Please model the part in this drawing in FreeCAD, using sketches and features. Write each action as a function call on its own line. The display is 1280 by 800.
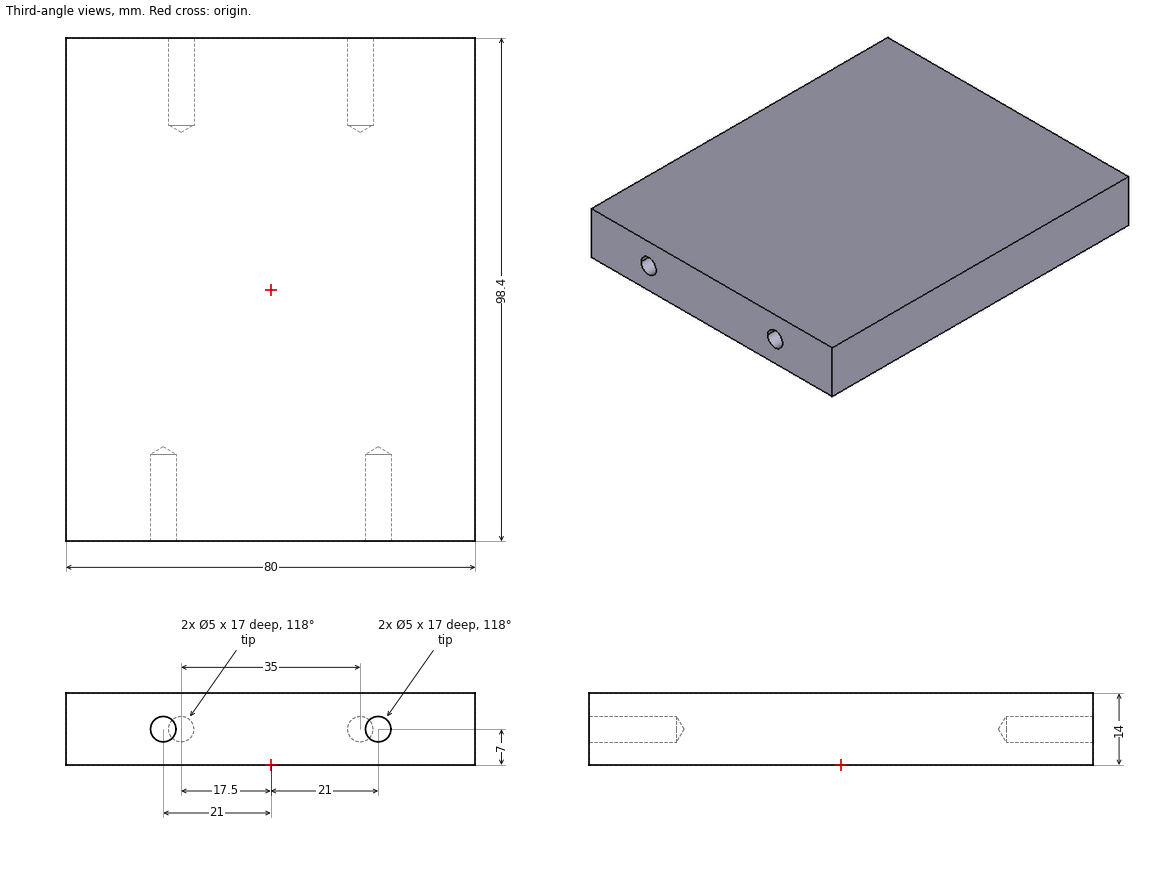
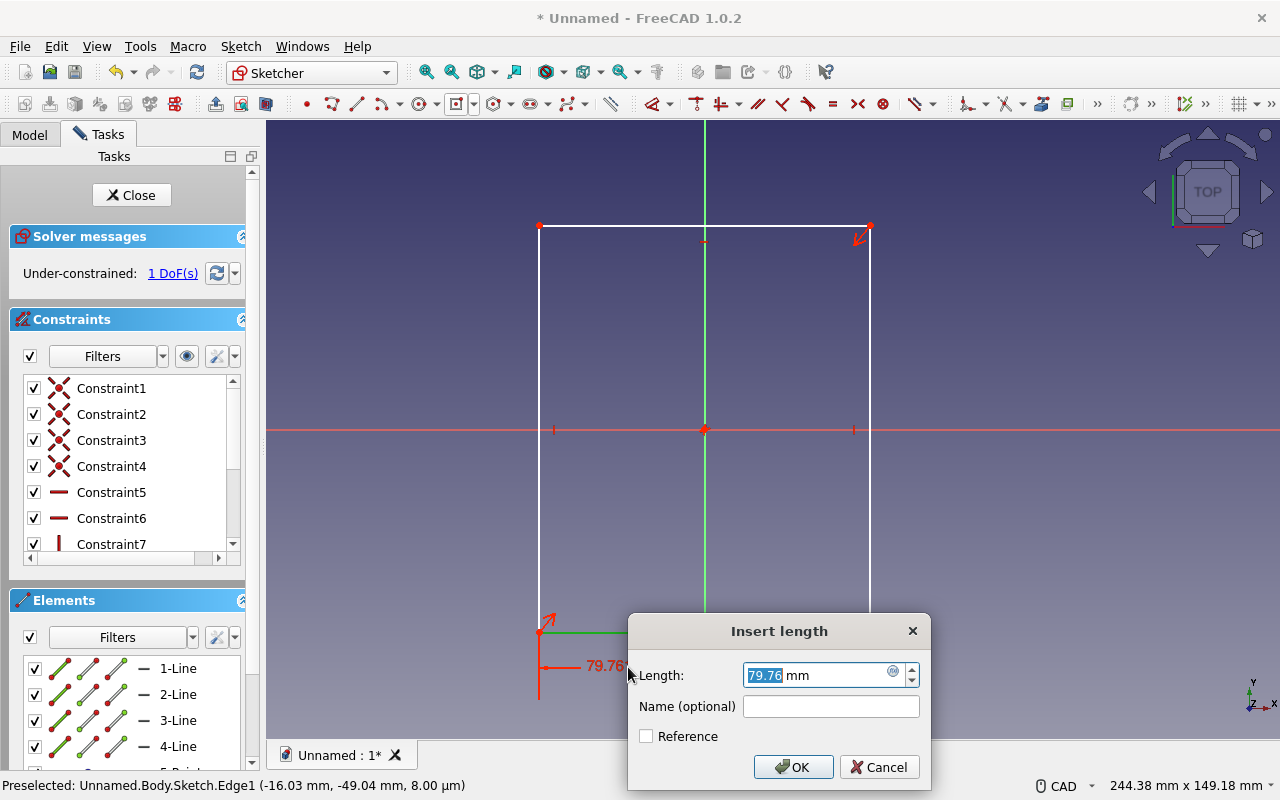
text(80)
key(Return)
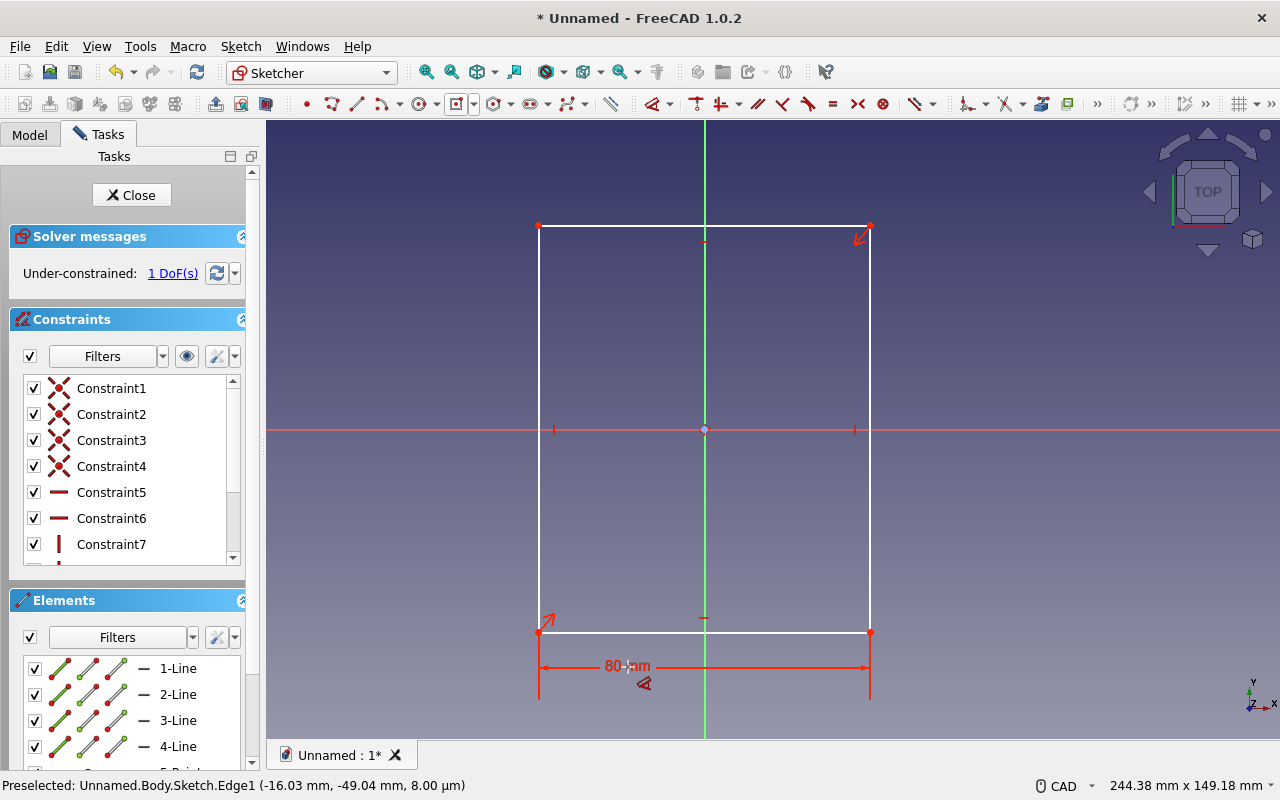
click(870, 511)
click(904, 336)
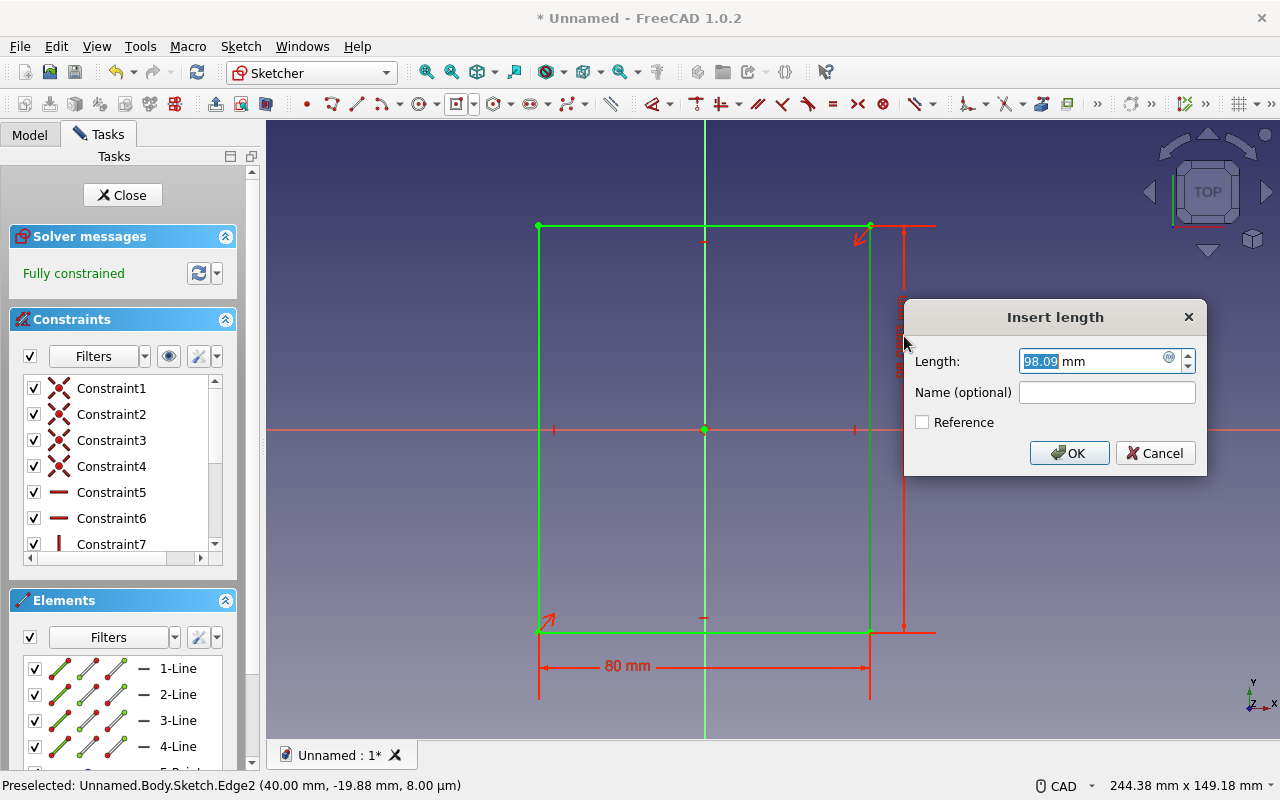
text(98.4)
key(Return)
key(Escape)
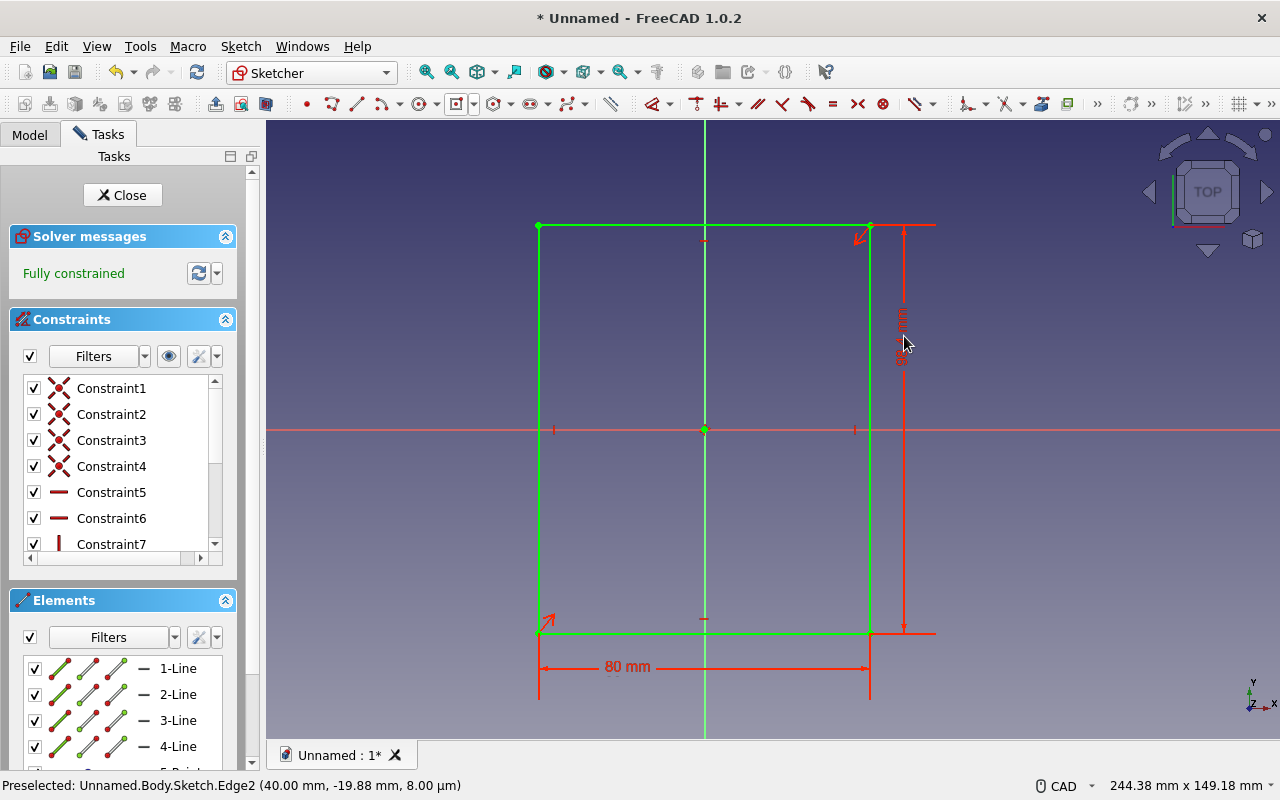
click(123, 195)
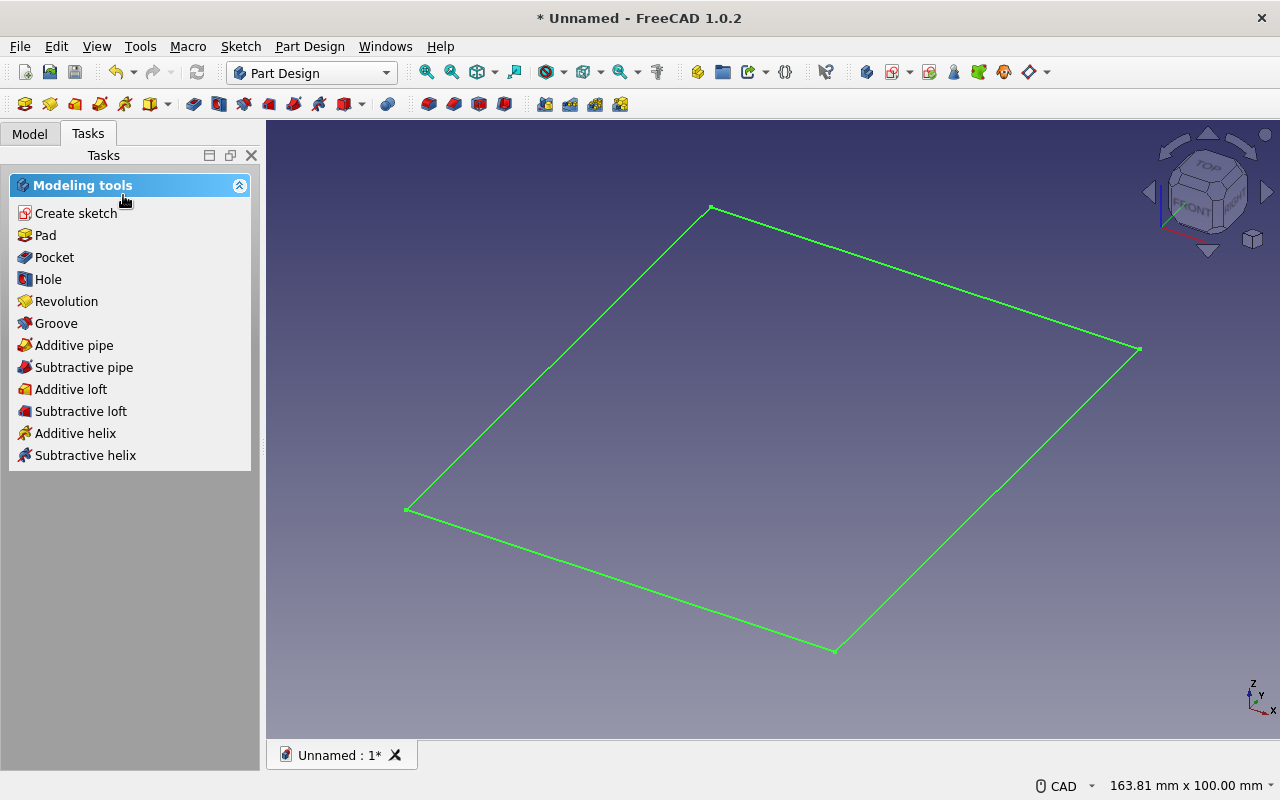
click(25, 104)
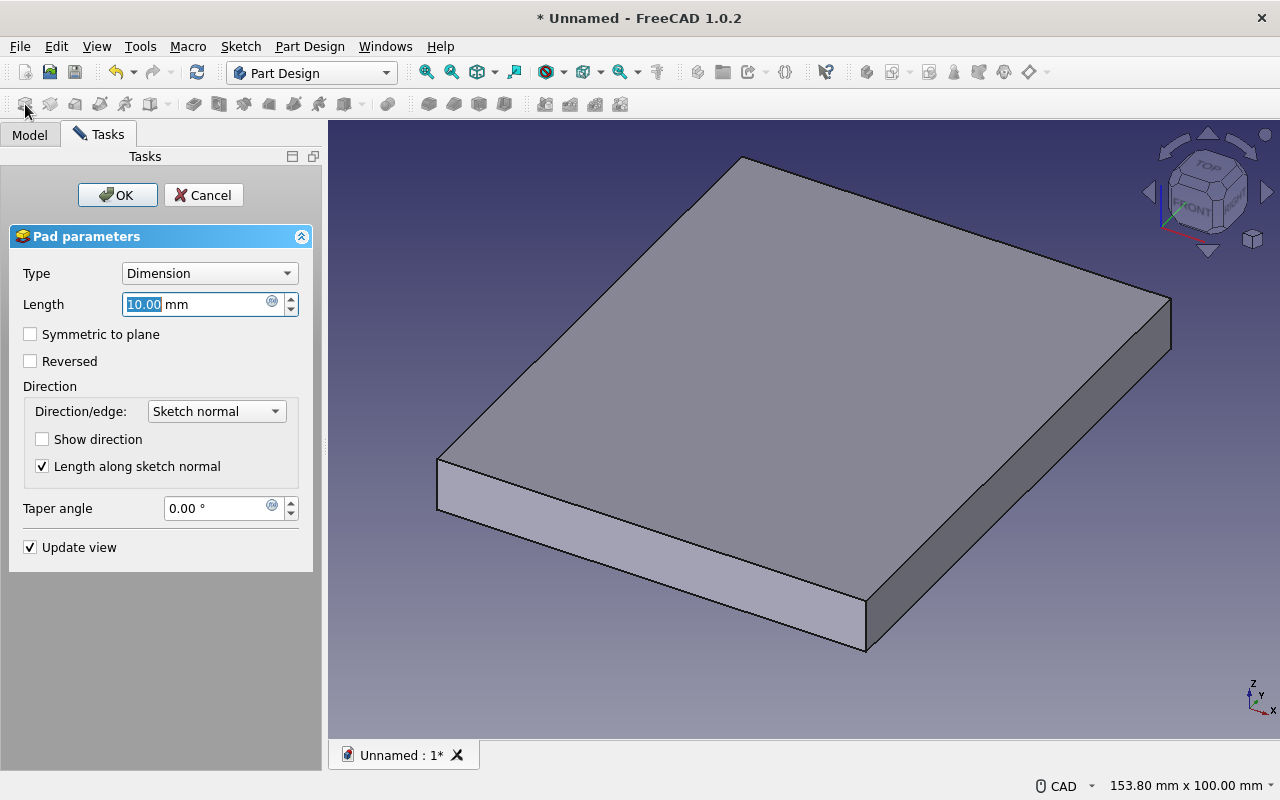
text(14)
key(Tab)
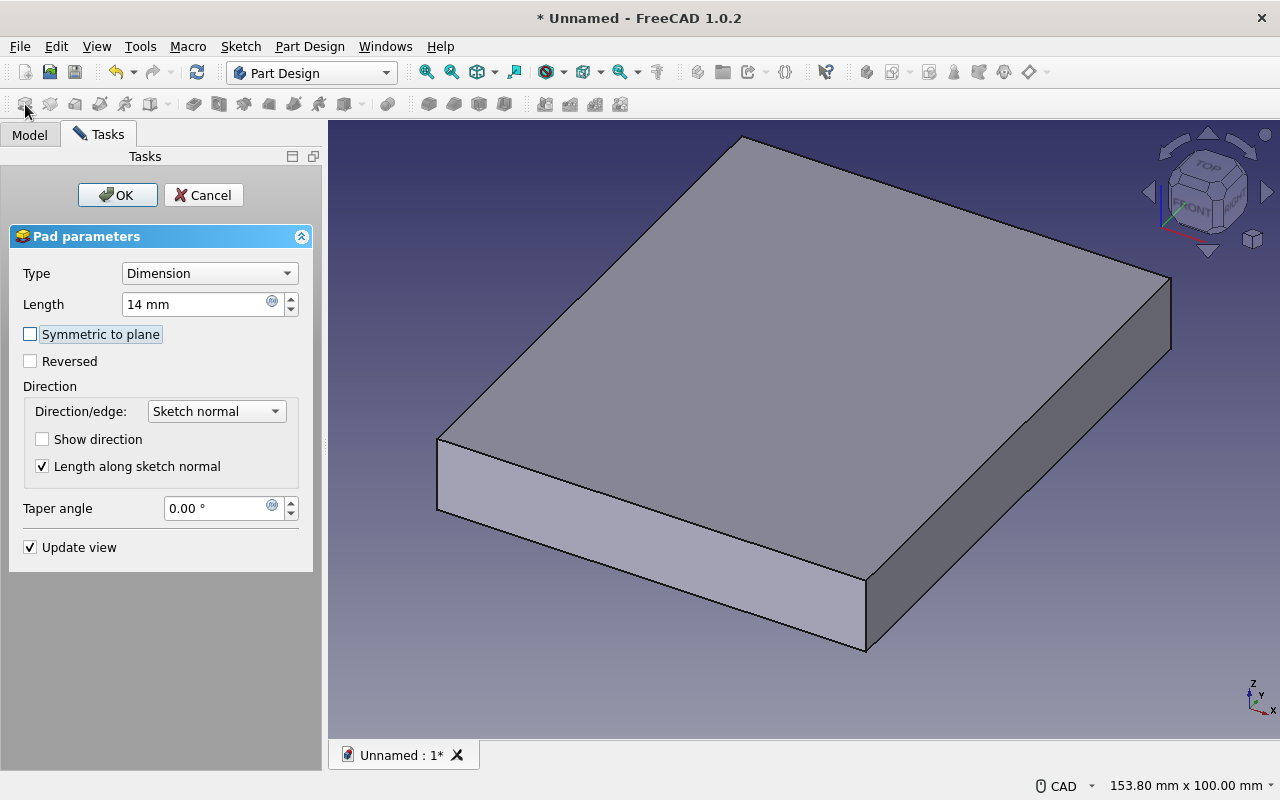
click(118, 195)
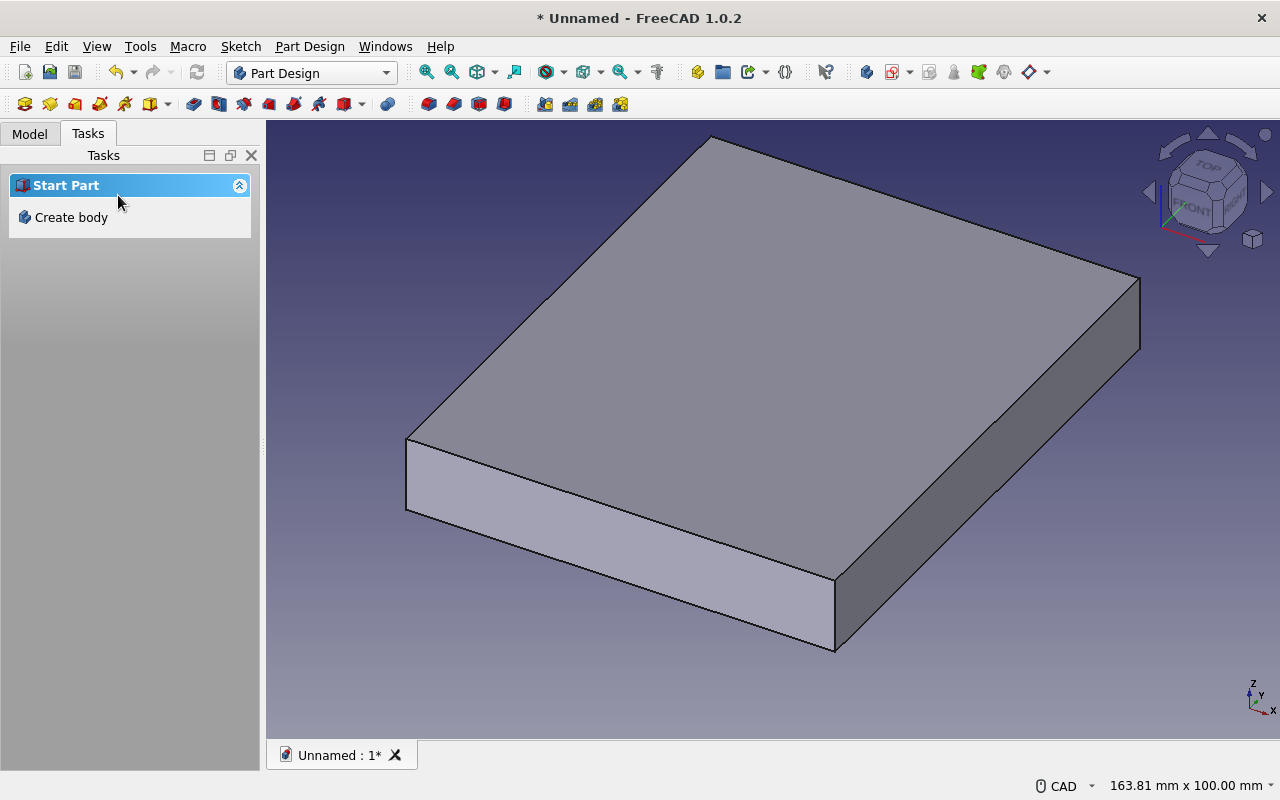
click(743, 585)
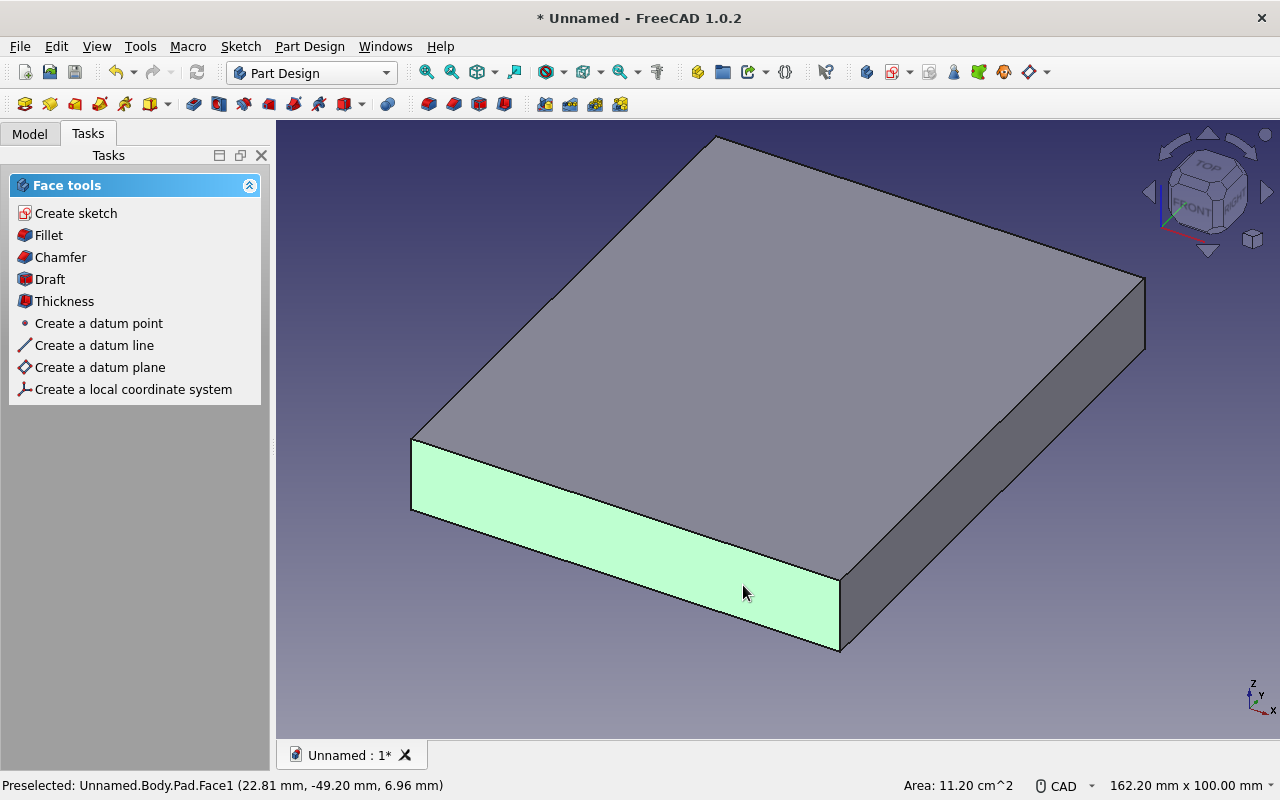
click(892, 72)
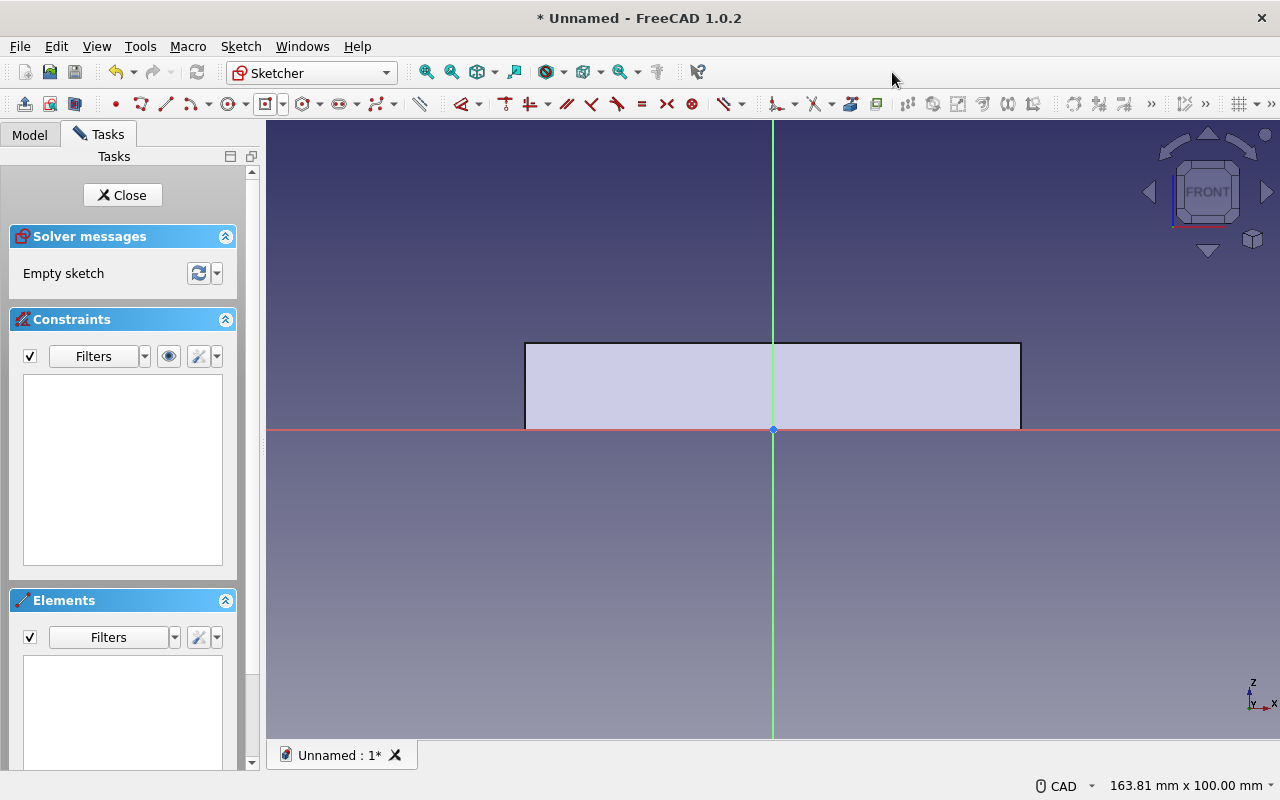
scroll(856, 364, up, 3)